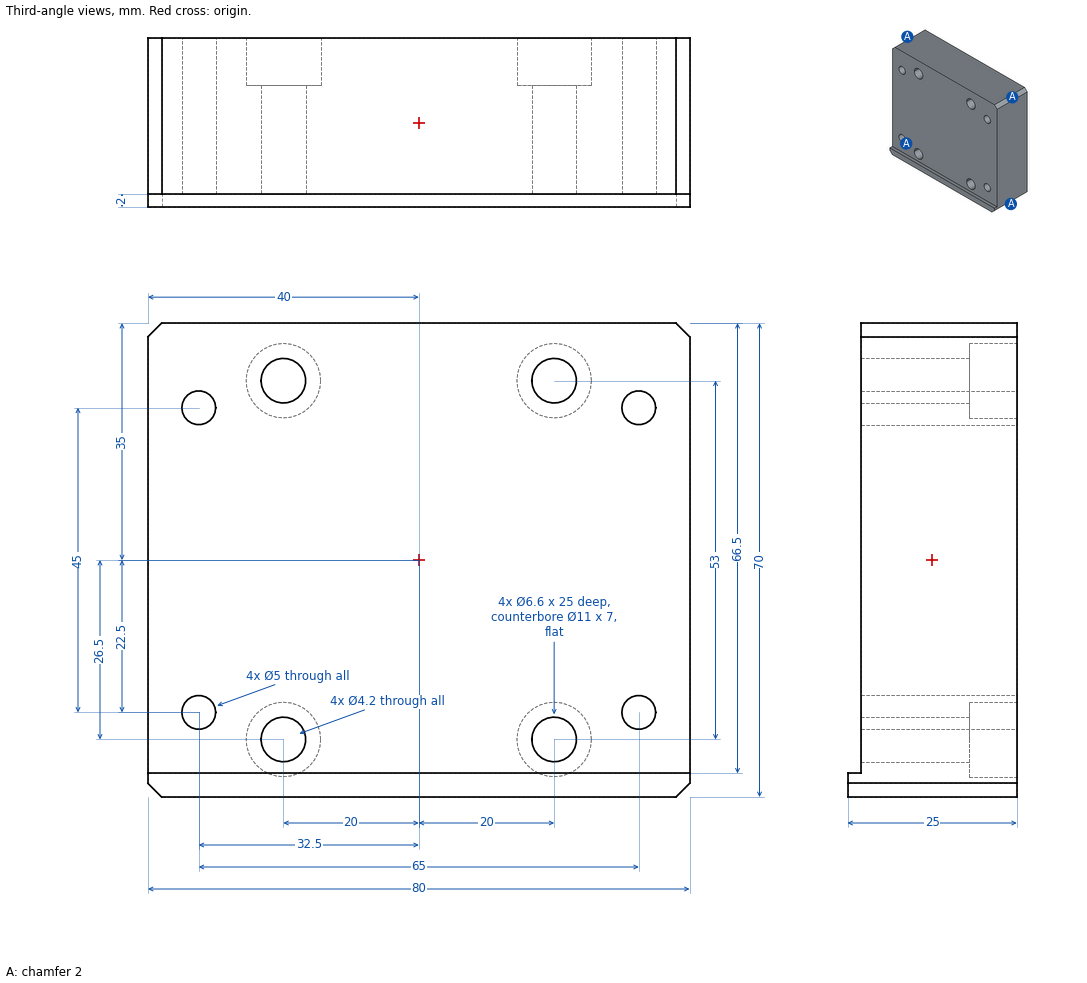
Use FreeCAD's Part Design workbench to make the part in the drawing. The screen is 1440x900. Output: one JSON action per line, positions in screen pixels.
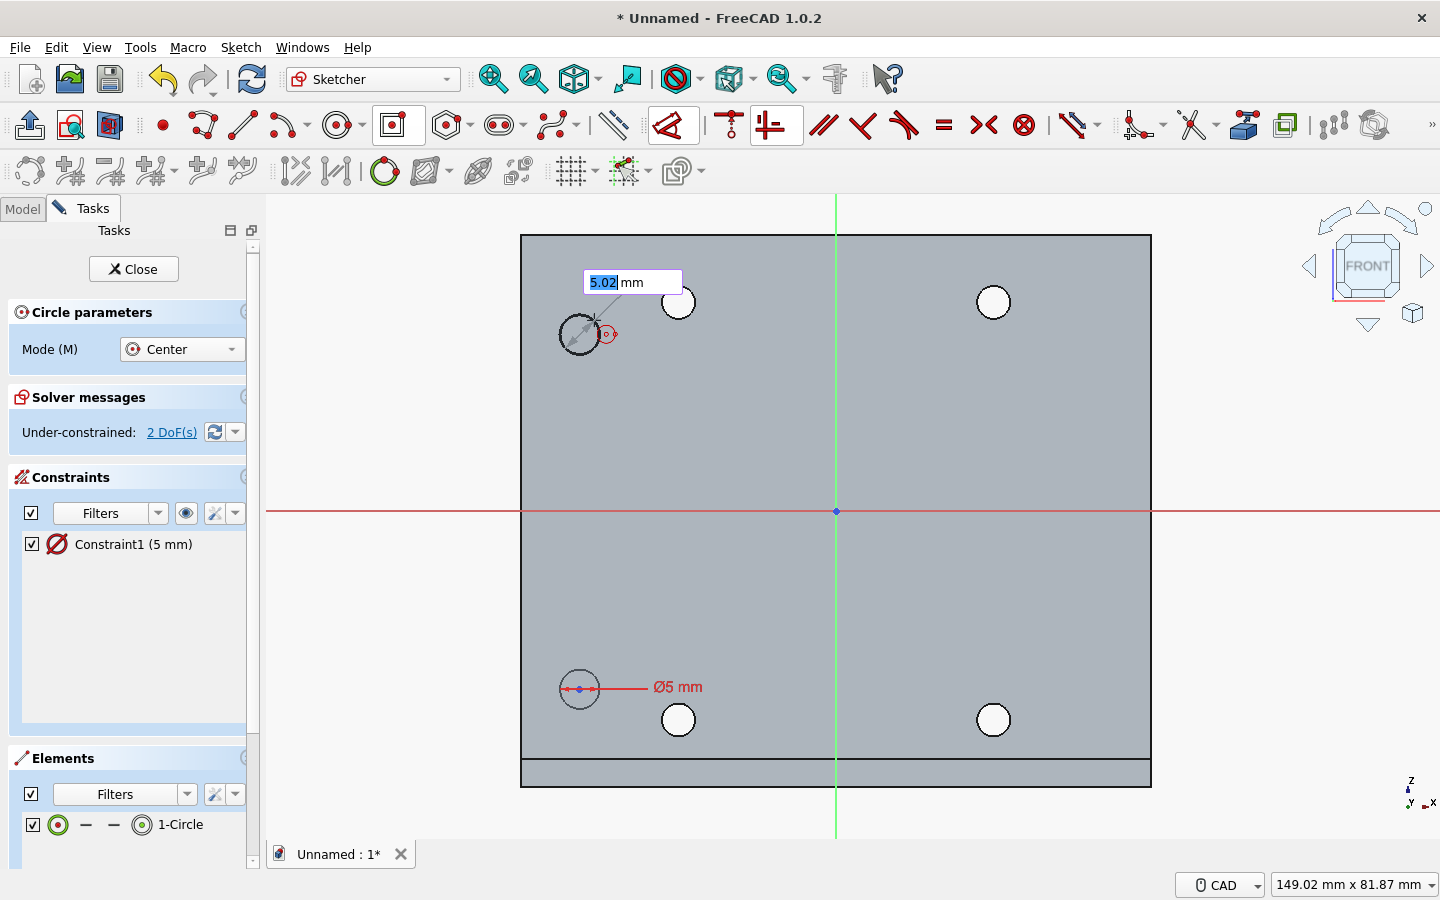
{"action": "type", "text": "5"}
{"action": "key", "text": "Return"}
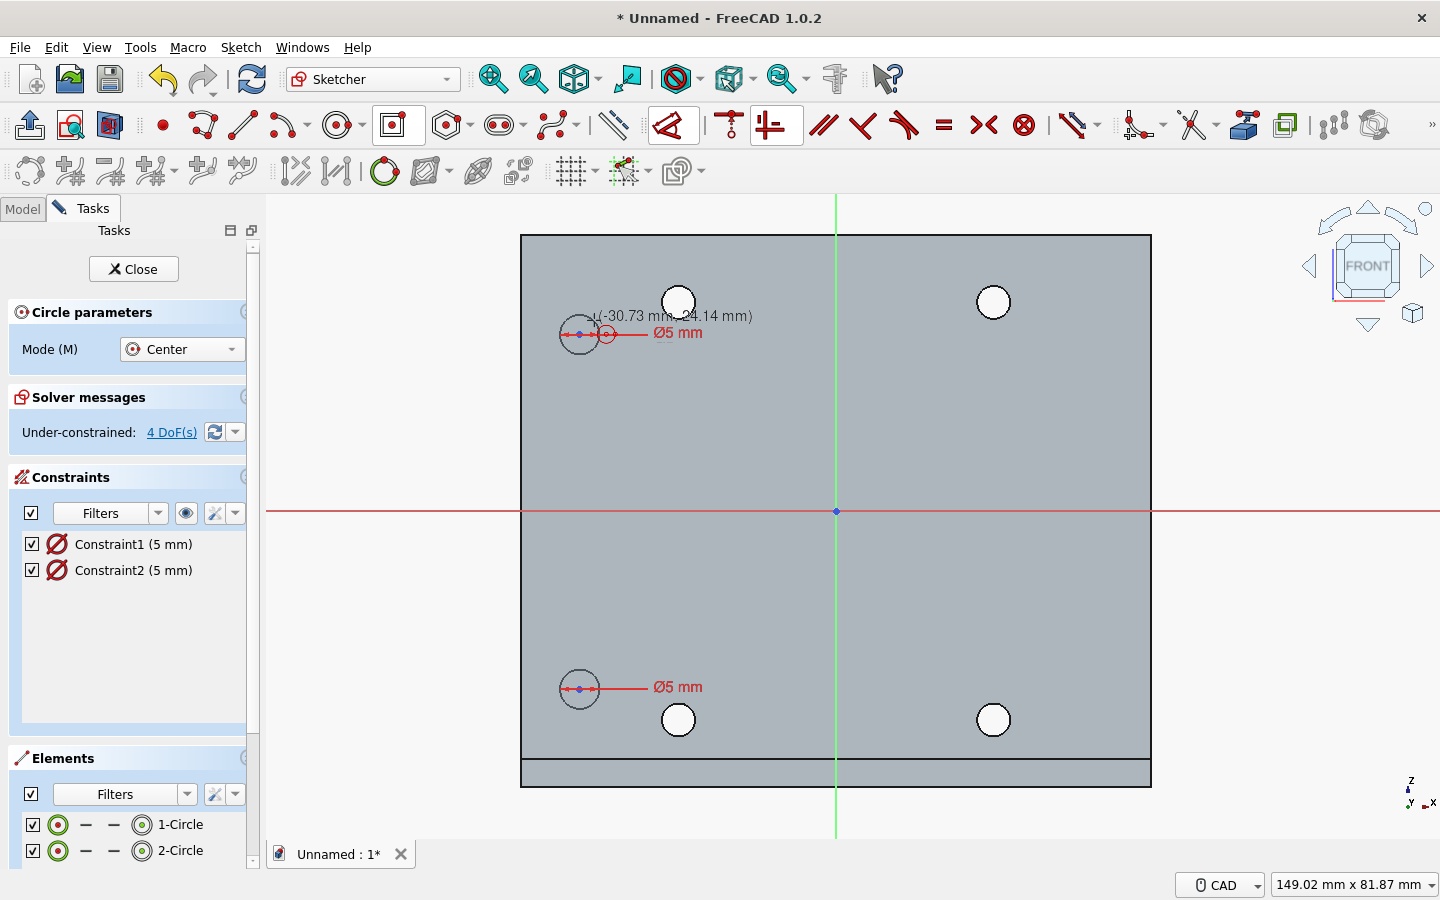
{"action": "left_click", "coordinate": [1092, 688]}
{"action": "mouse_move", "coordinate": [1106, 675]}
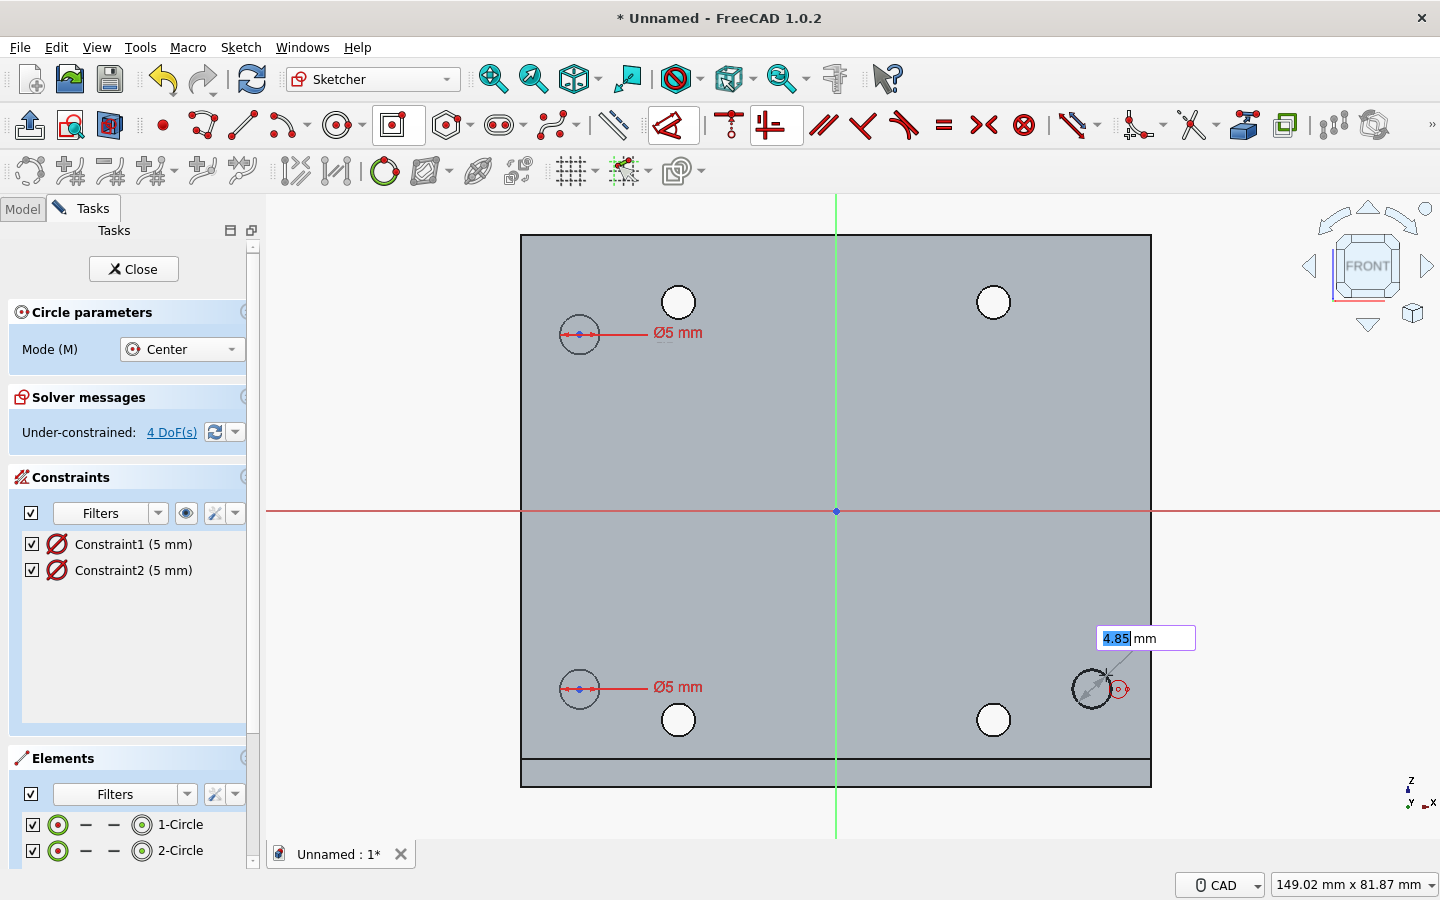
{"action": "type", "text": "5"}
{"action": "key", "text": "Return"}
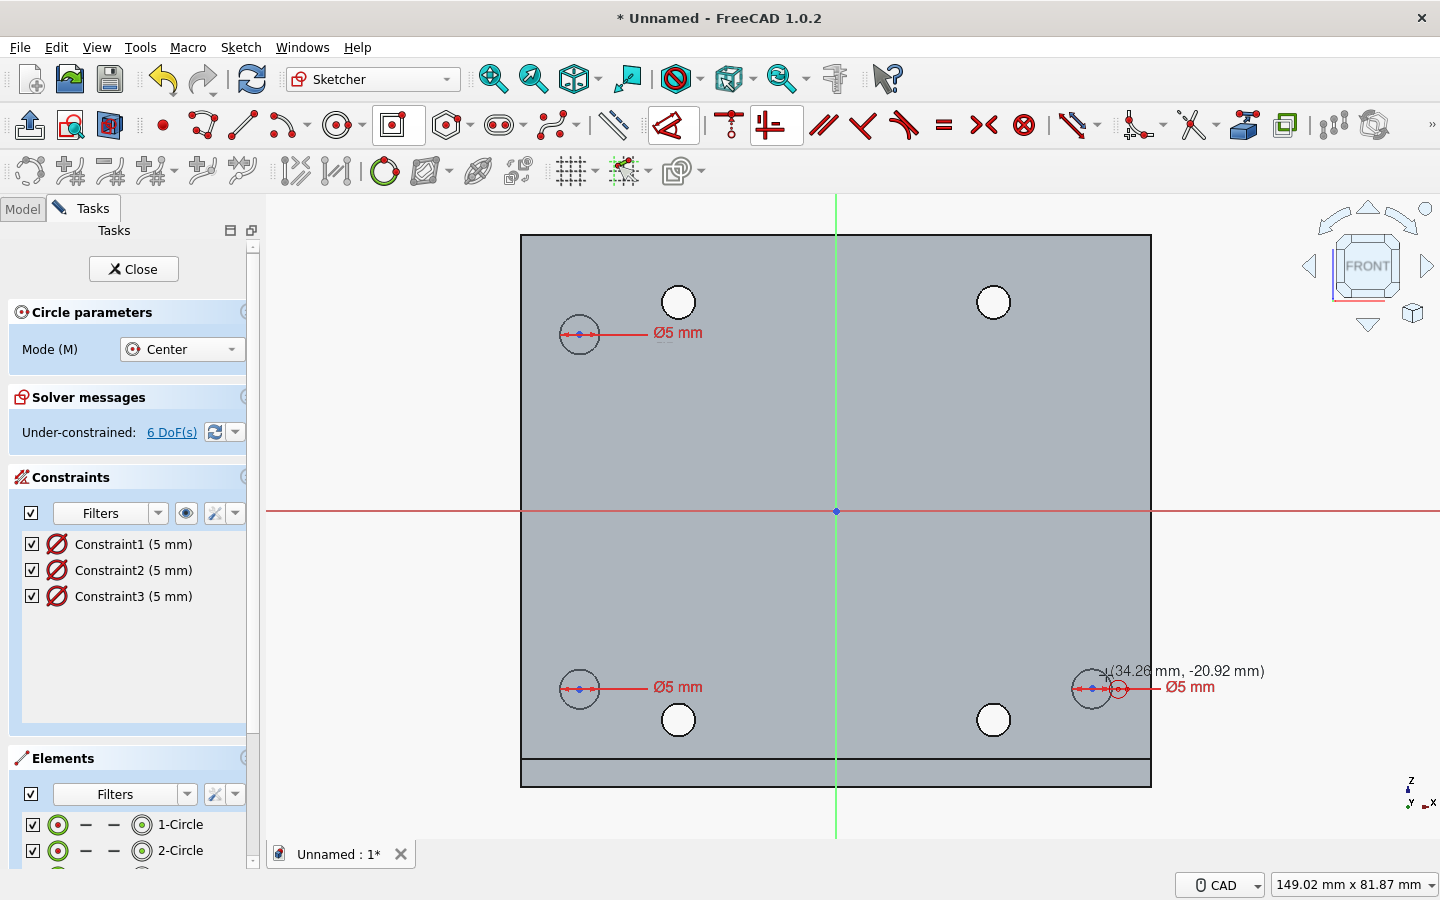
{"action": "left_click", "coordinate": [1092, 334]}
{"action": "mouse_move", "coordinate": [1106, 320]}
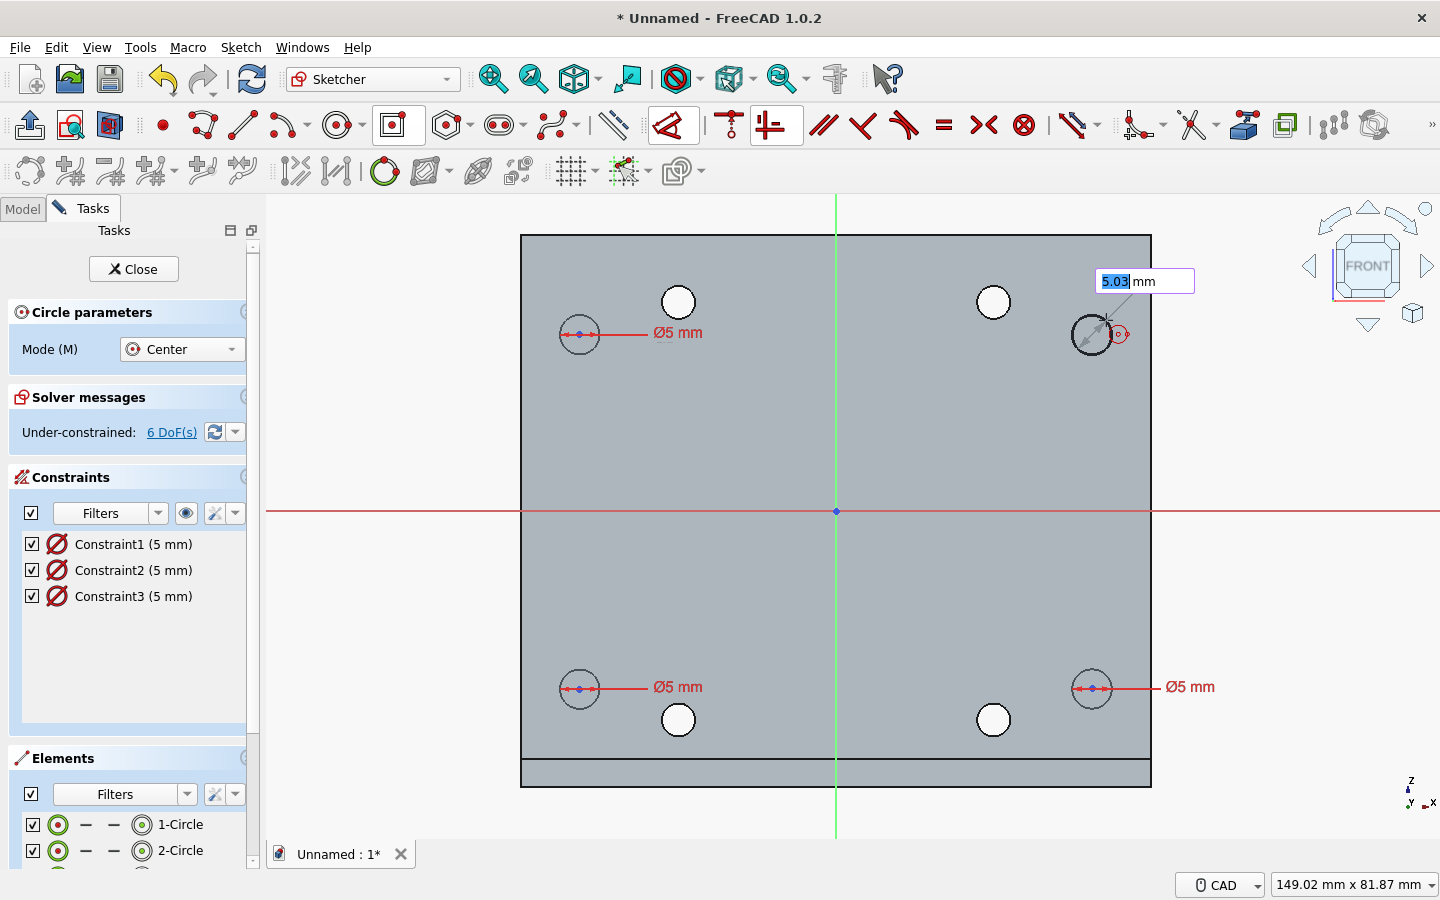
{"action": "type", "text": "5"}
{"action": "key", "text": "Return"}
{"action": "key", "text": "Escape"}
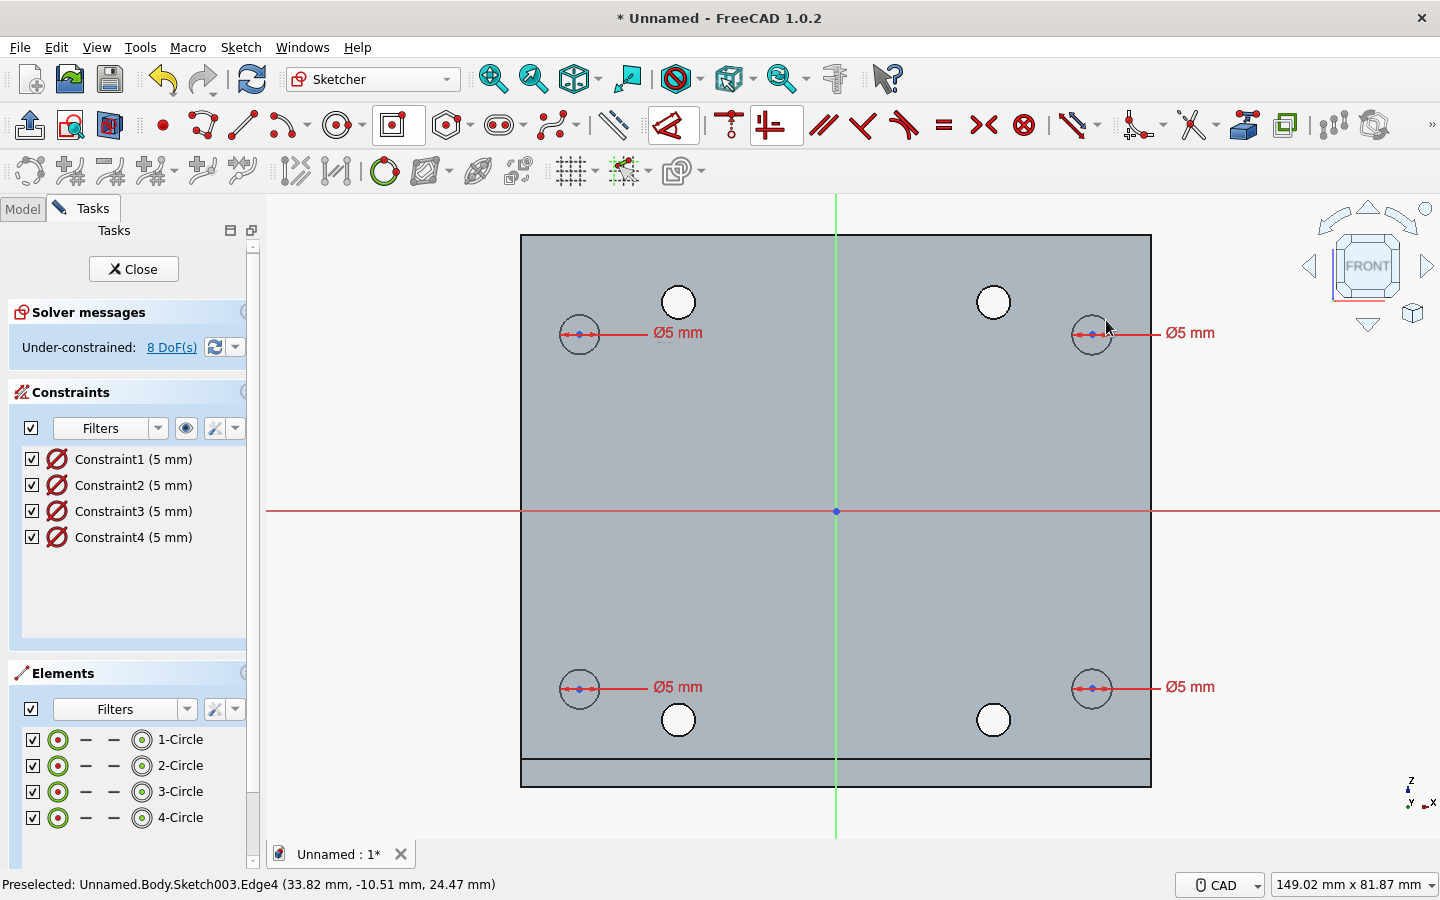
{"action": "left_click", "coordinate": [580, 689]}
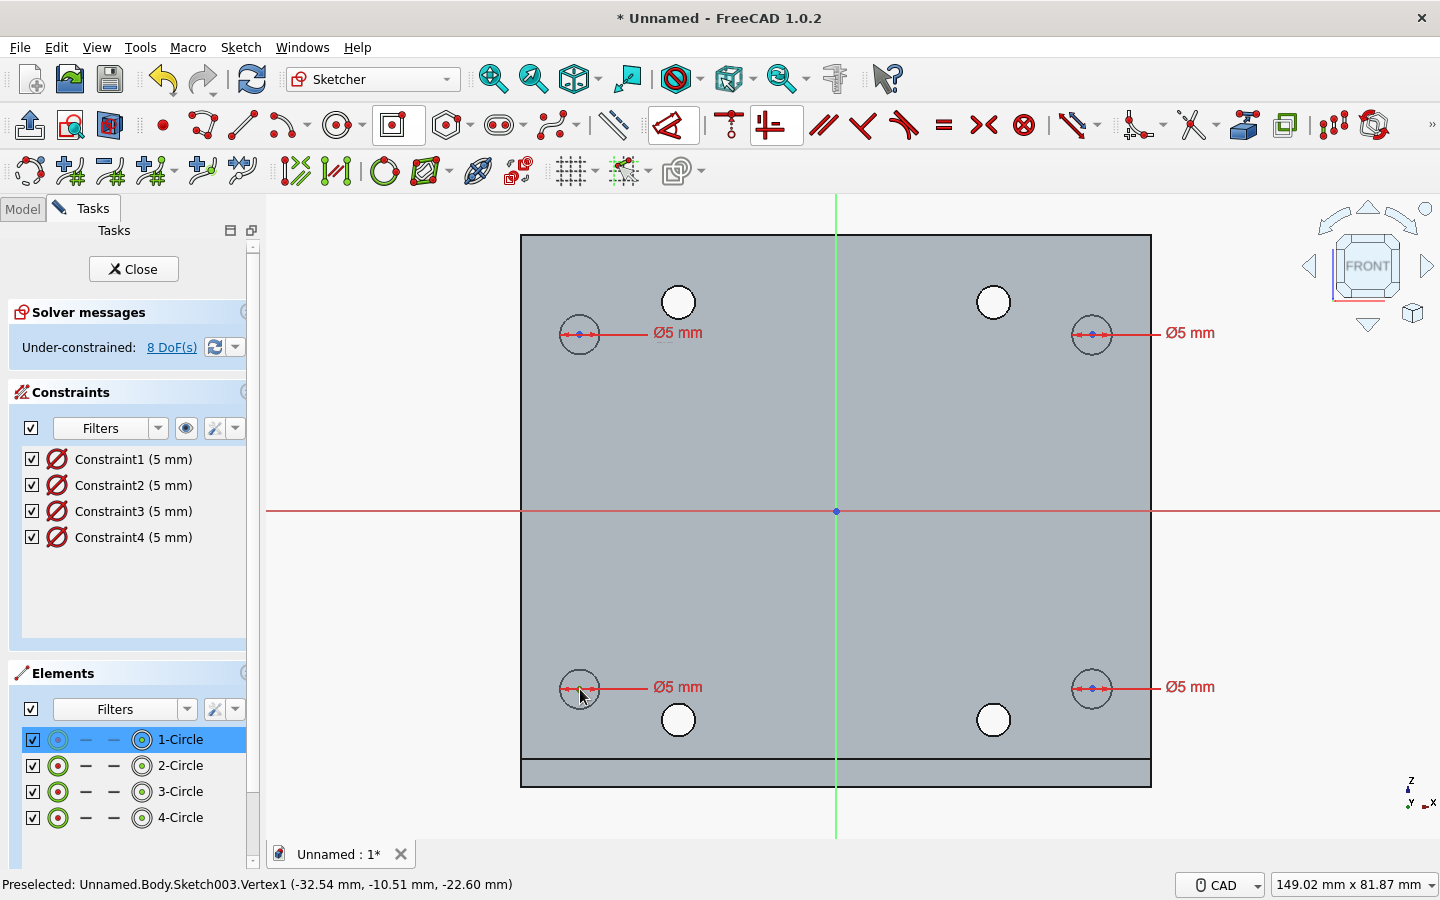
{"action": "left_click", "coordinate": [580, 335]}